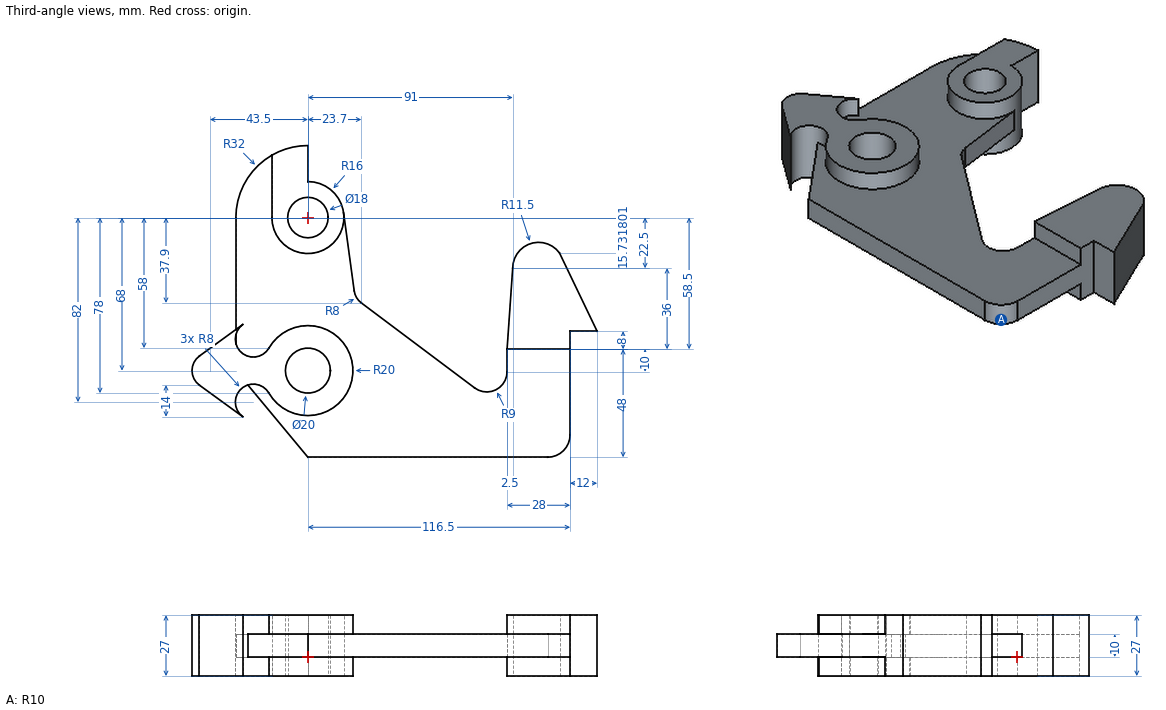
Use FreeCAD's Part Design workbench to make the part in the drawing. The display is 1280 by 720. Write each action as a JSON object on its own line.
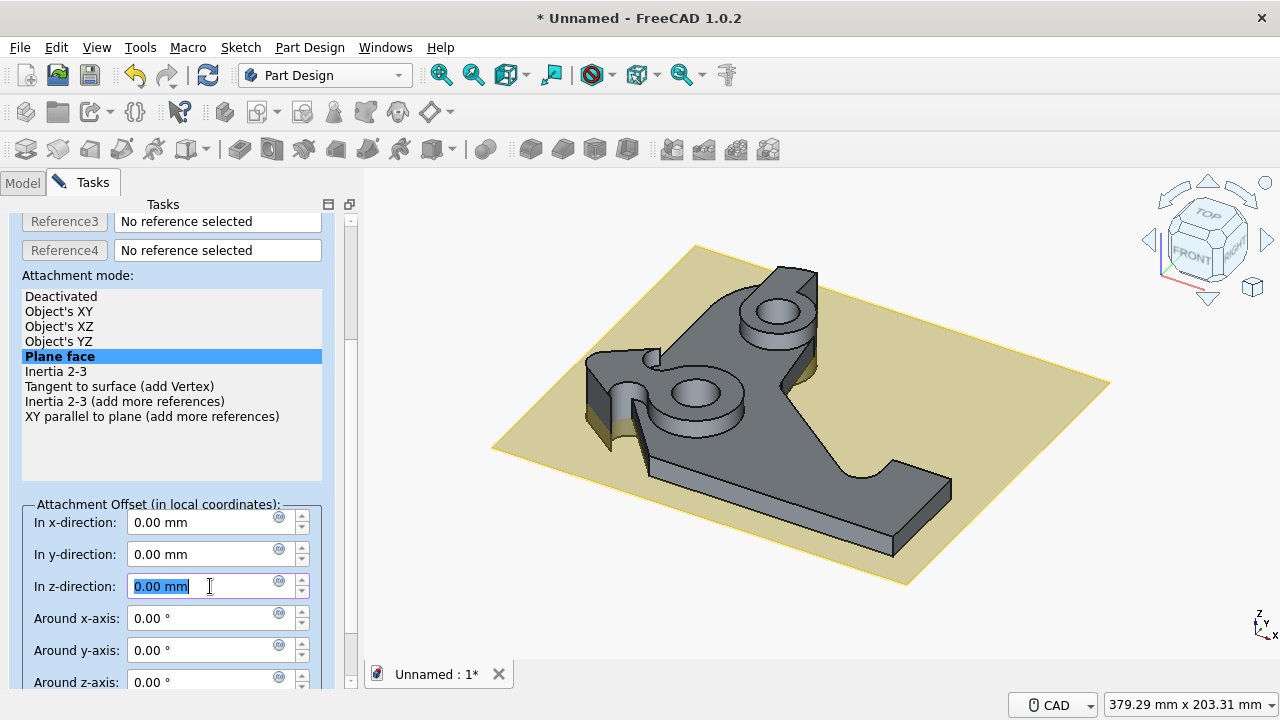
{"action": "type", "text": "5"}
{"action": "key", "text": "Tab"}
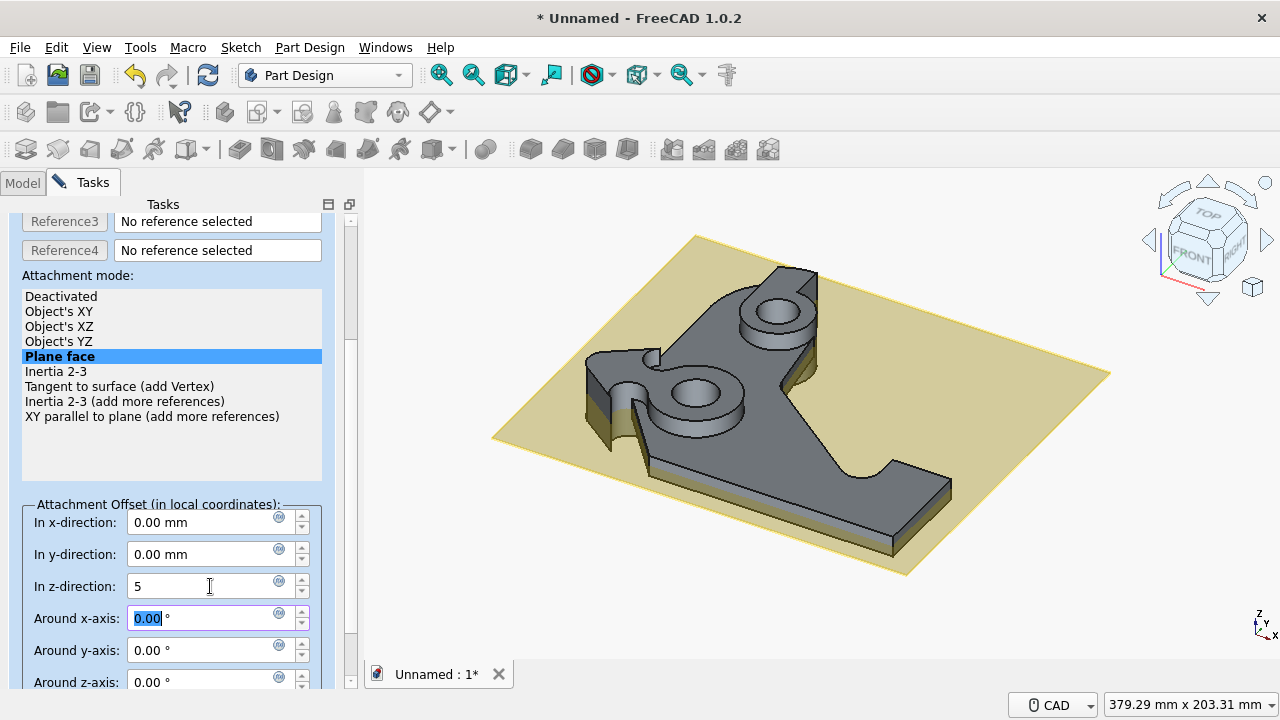
{"action": "scroll", "coordinate": [351, 451], "scroll_direction": "up", "scroll_amount": 4}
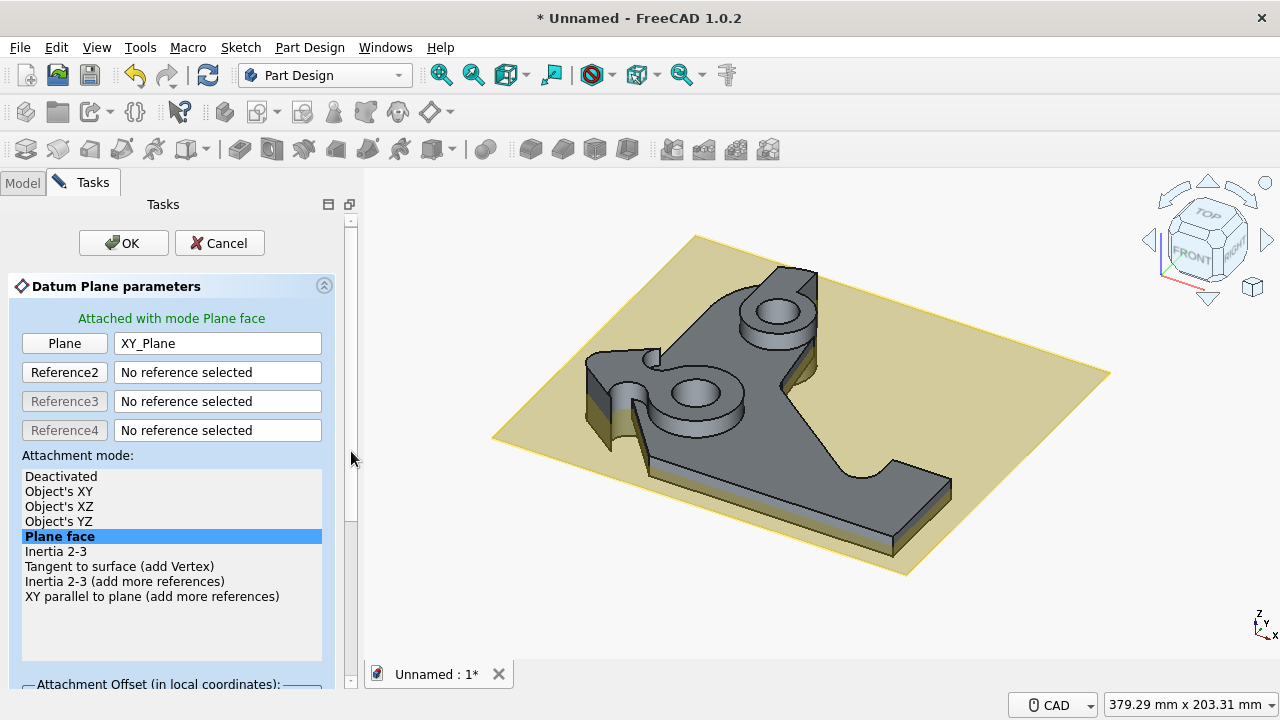
{"action": "left_click", "coordinate": [124, 243]}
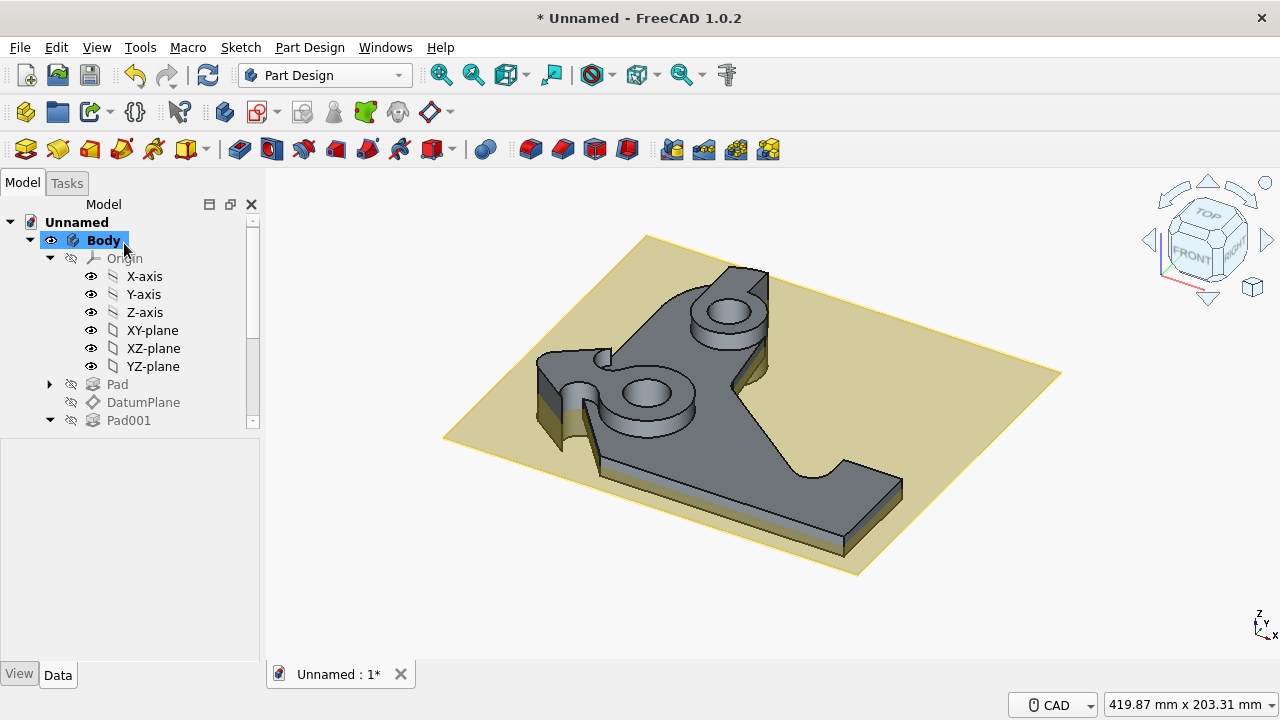
{"action": "scroll", "coordinate": [100, 326], "scroll_direction": "down", "scroll_amount": 3}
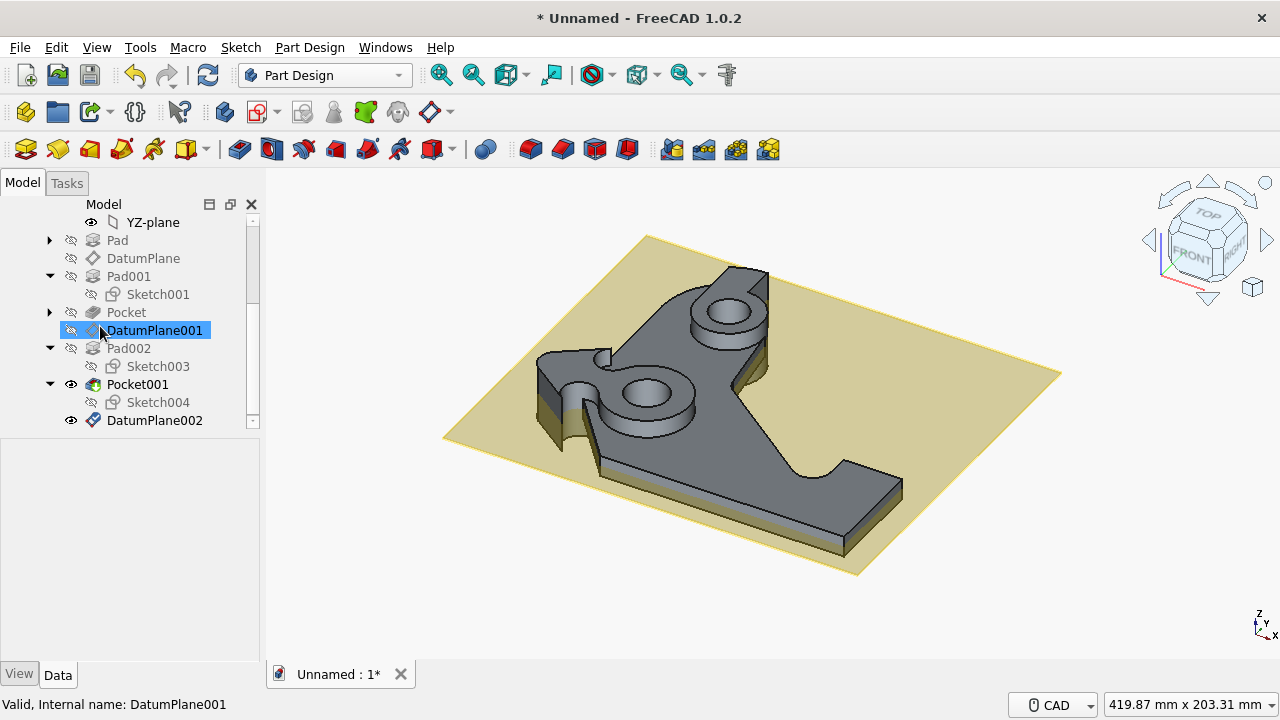
{"action": "left_click", "coordinate": [116, 420]}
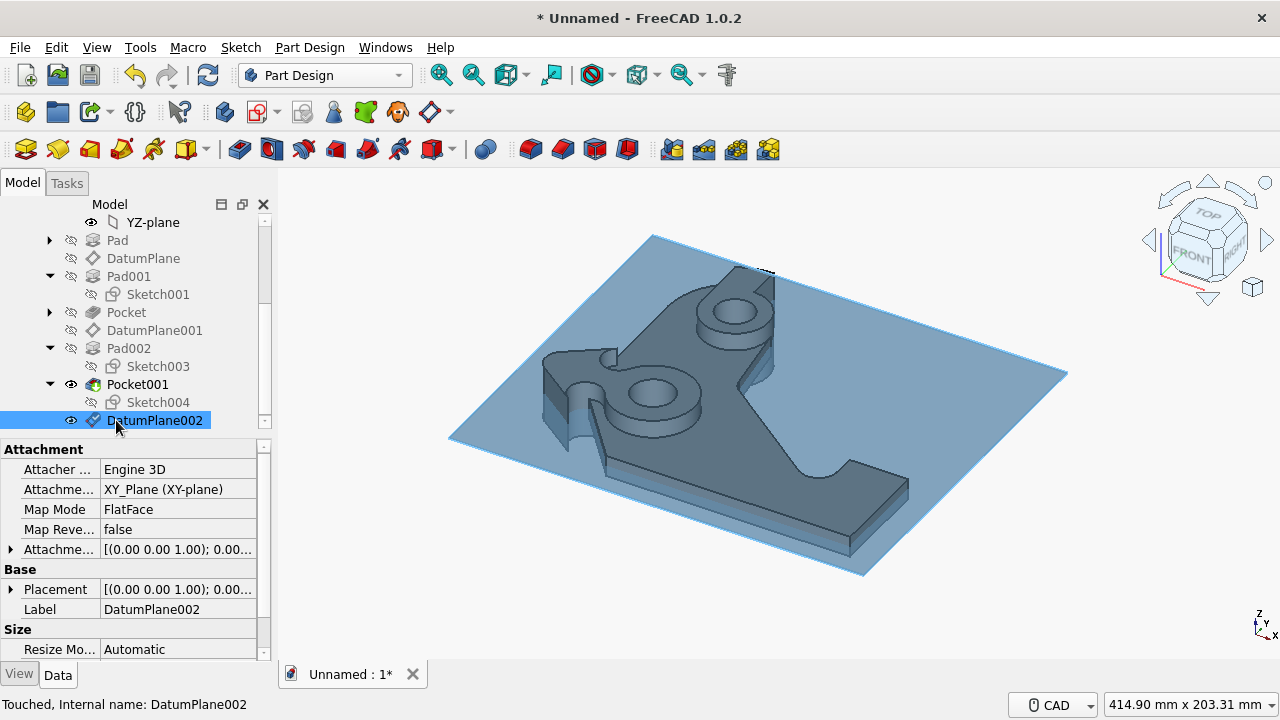
{"action": "left_click", "coordinate": [258, 112]}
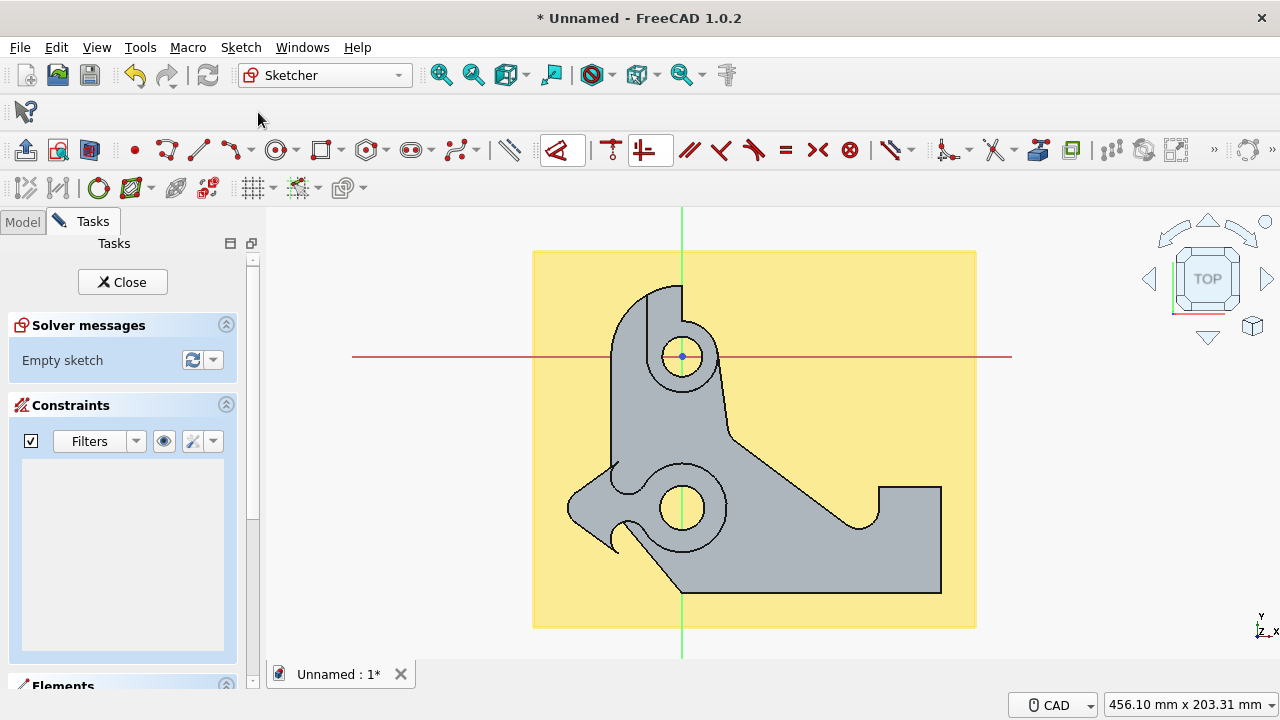
{"action": "left_click", "coordinate": [90, 150]}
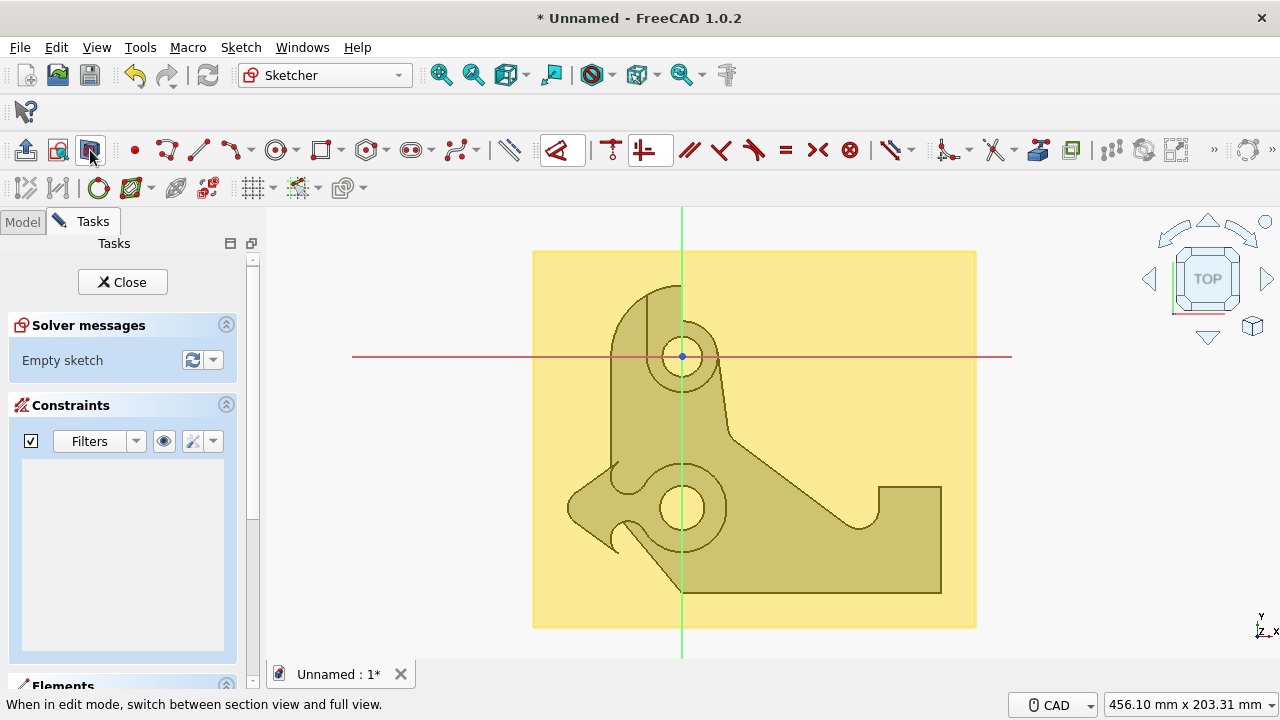
{"action": "scroll", "coordinate": [1051, 435], "scroll_direction": "up", "scroll_amount": 5}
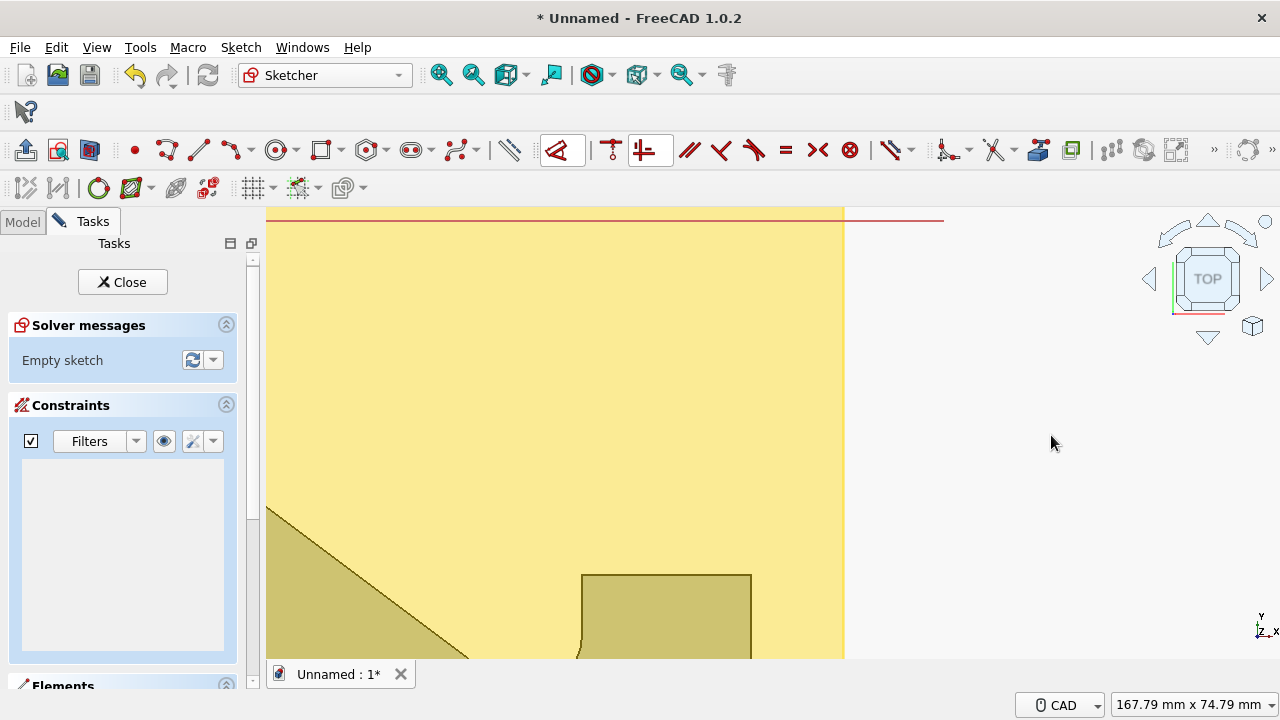
{"action": "key", "text": "g m"}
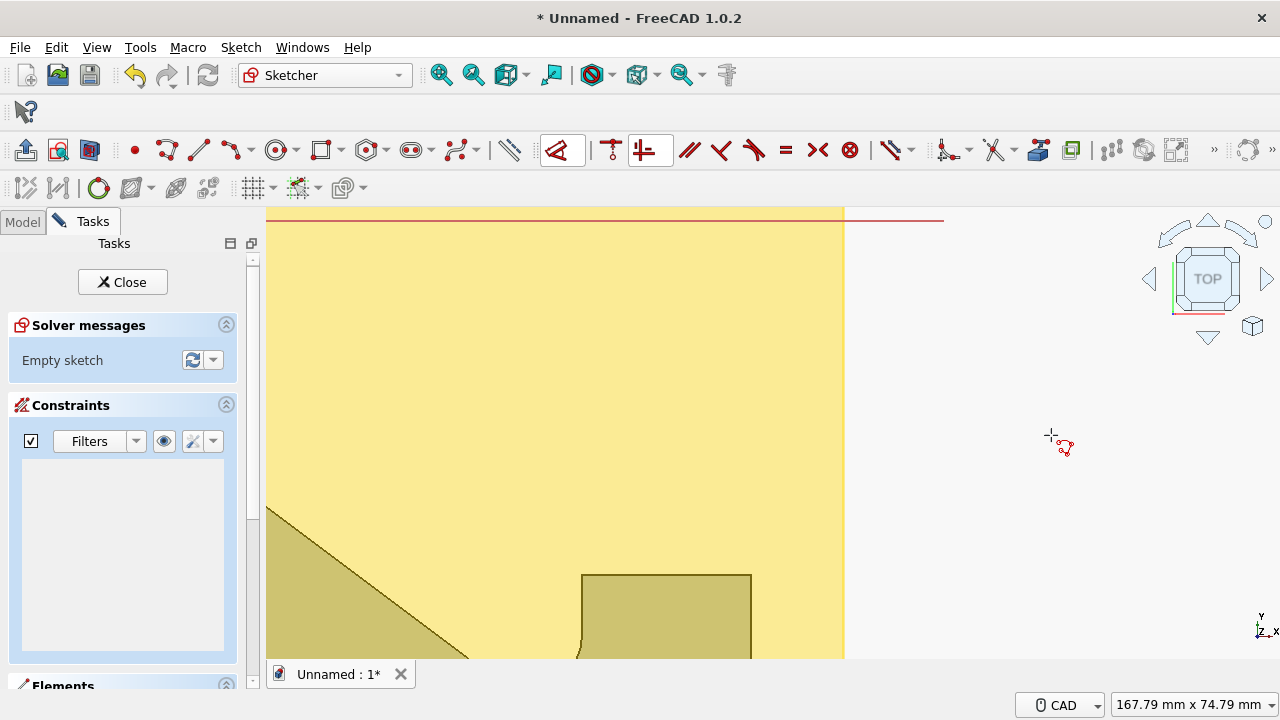
{"action": "left_click", "coordinate": [597, 357]}
{"action": "left_click", "coordinate": [582, 575]}
{"action": "left_click", "coordinate": [751, 575]}
{"action": "left_click", "coordinate": [751, 526]}
{"action": "left_click", "coordinate": [824, 526]}
{"action": "left_click", "coordinate": [723, 316]}
{"action": "right_click", "coordinate": [723, 316]}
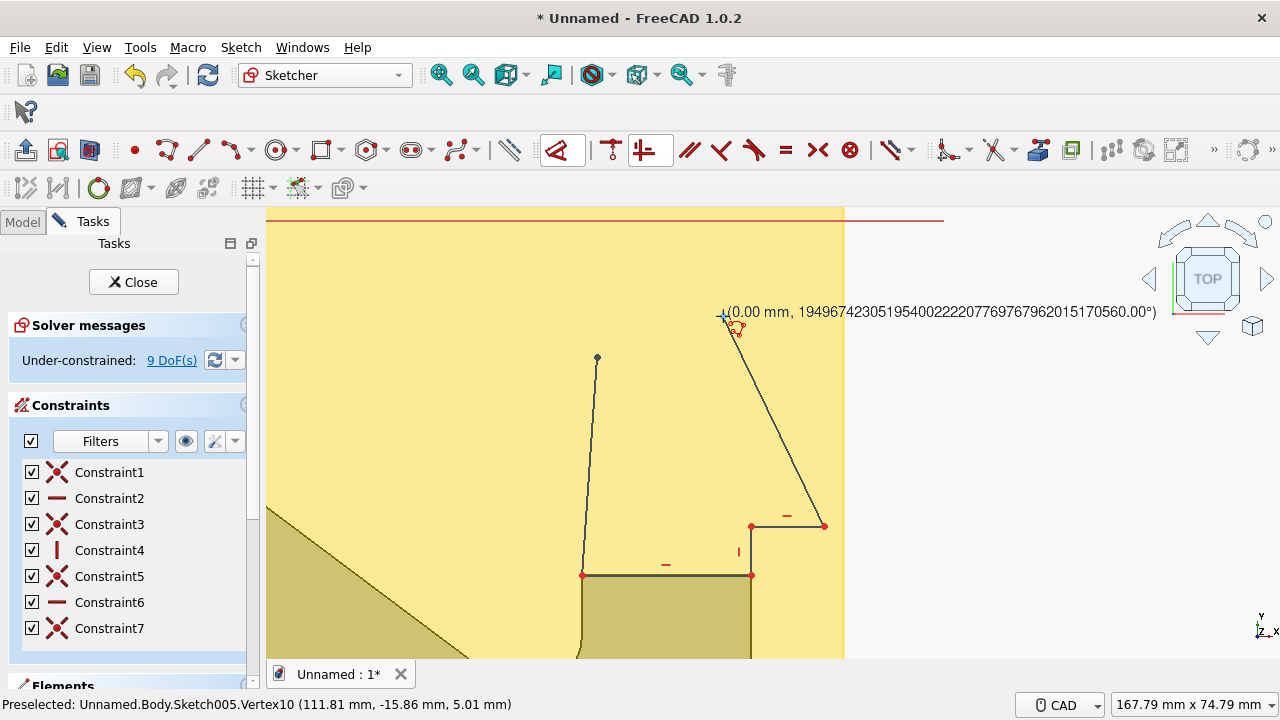
{"action": "left_click", "coordinate": [232, 150]}